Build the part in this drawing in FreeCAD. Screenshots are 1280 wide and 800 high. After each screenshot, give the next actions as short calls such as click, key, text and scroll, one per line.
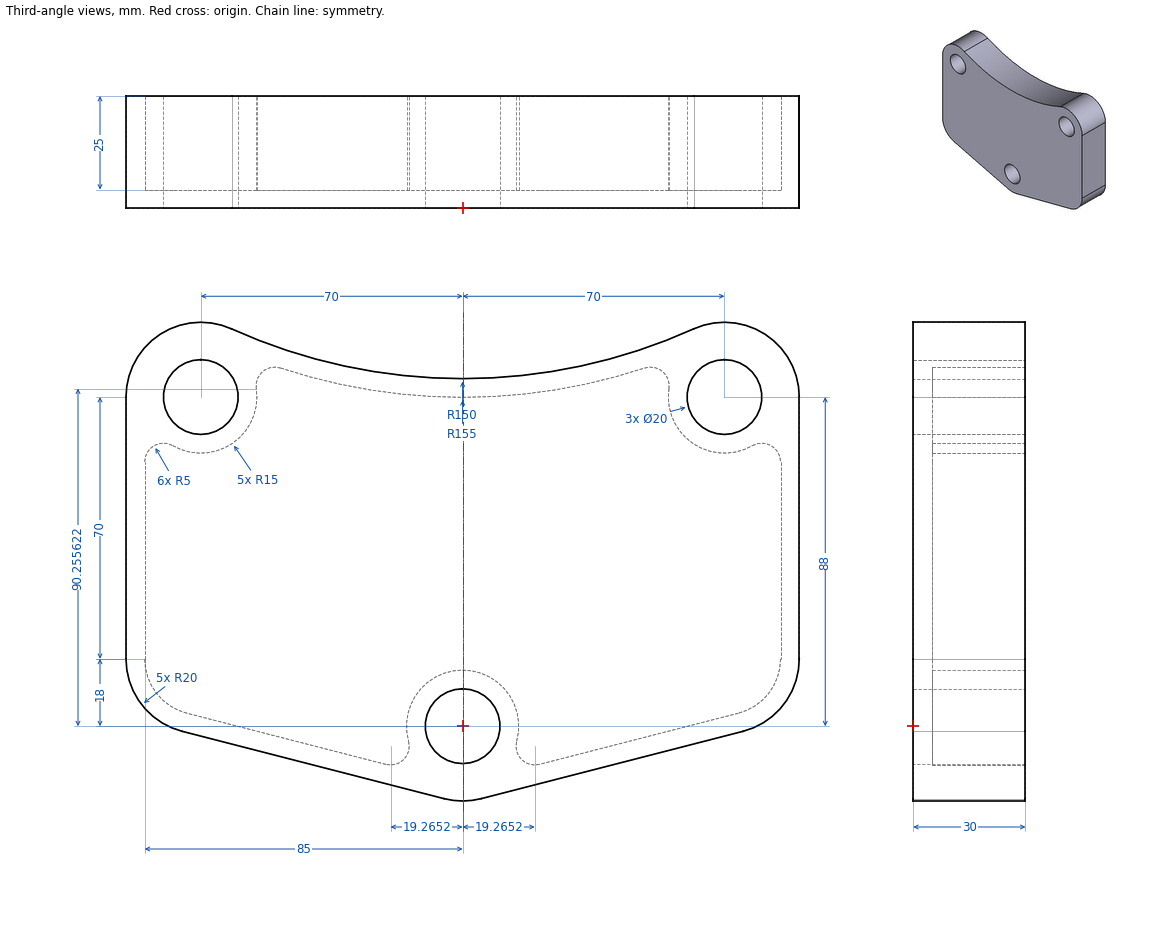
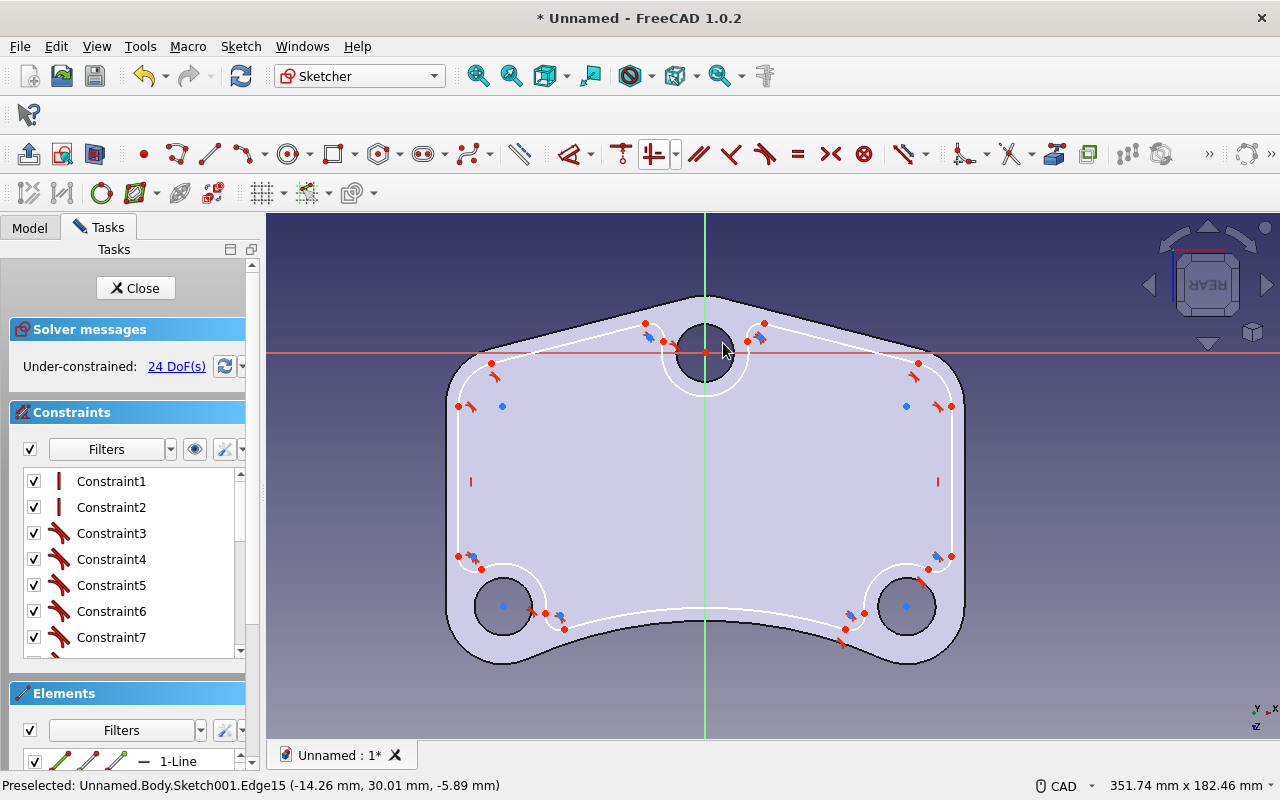
scroll(461, 565, up, 2)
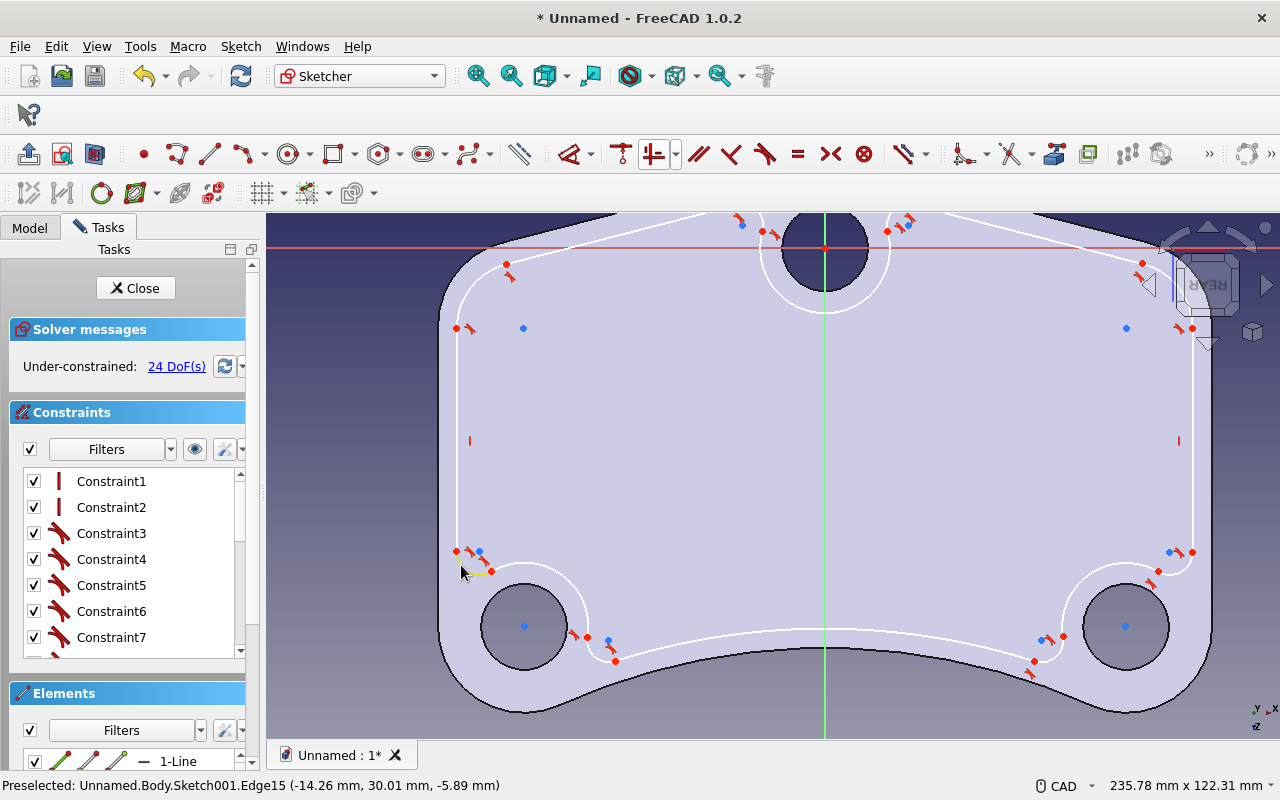
click(461, 565)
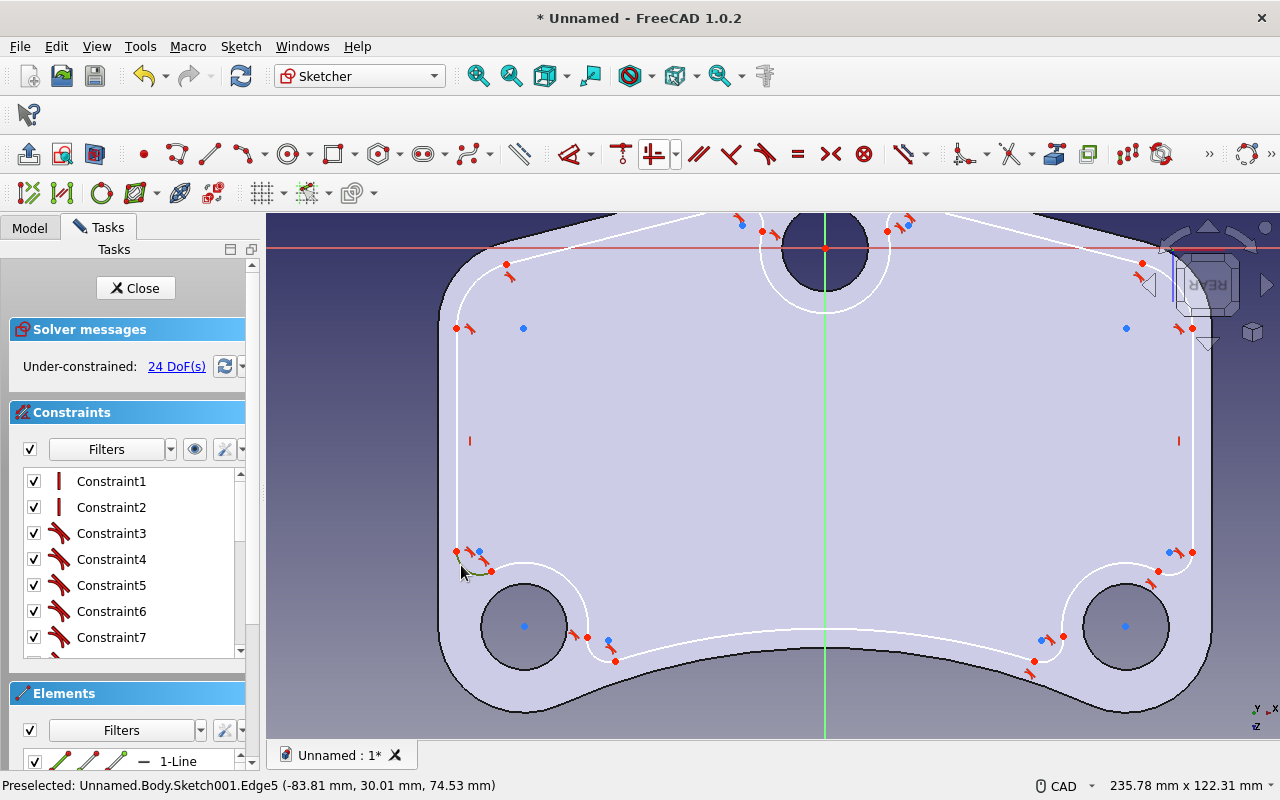
click(589, 650)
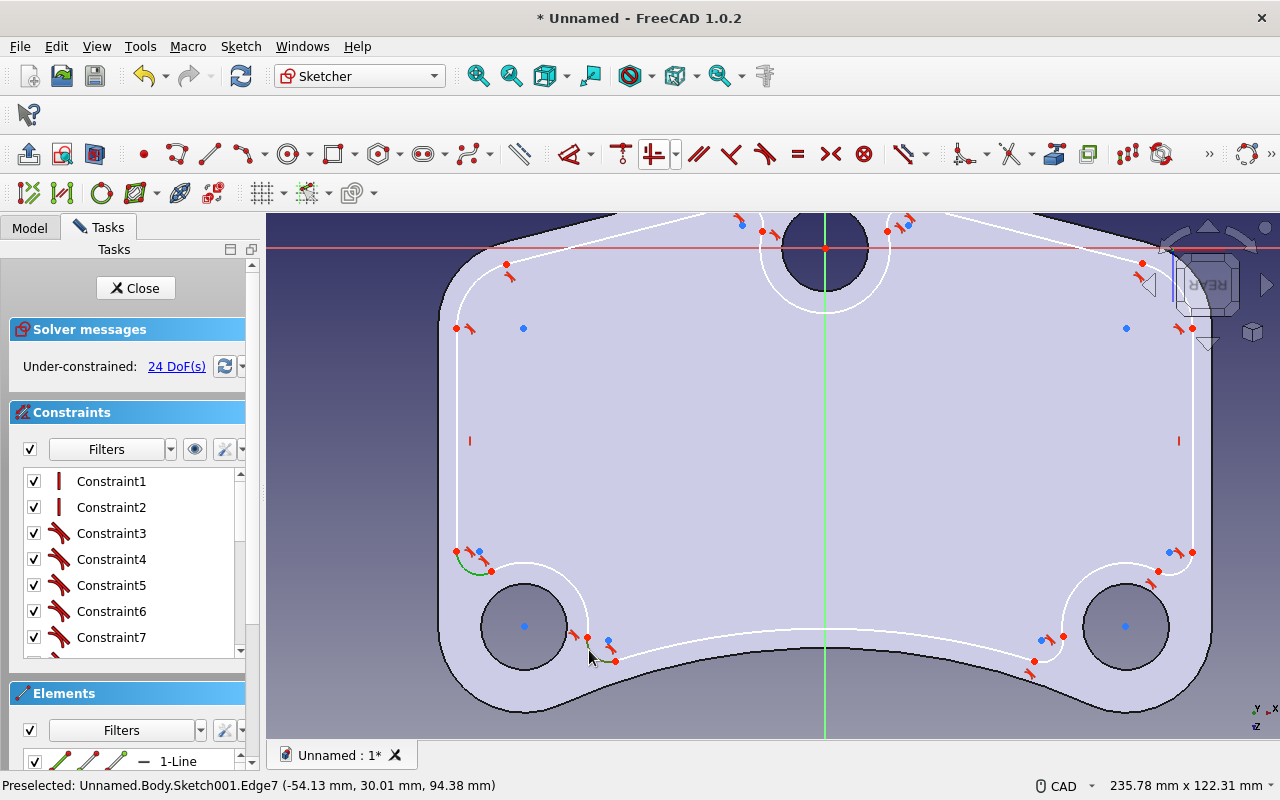
click(1048, 661)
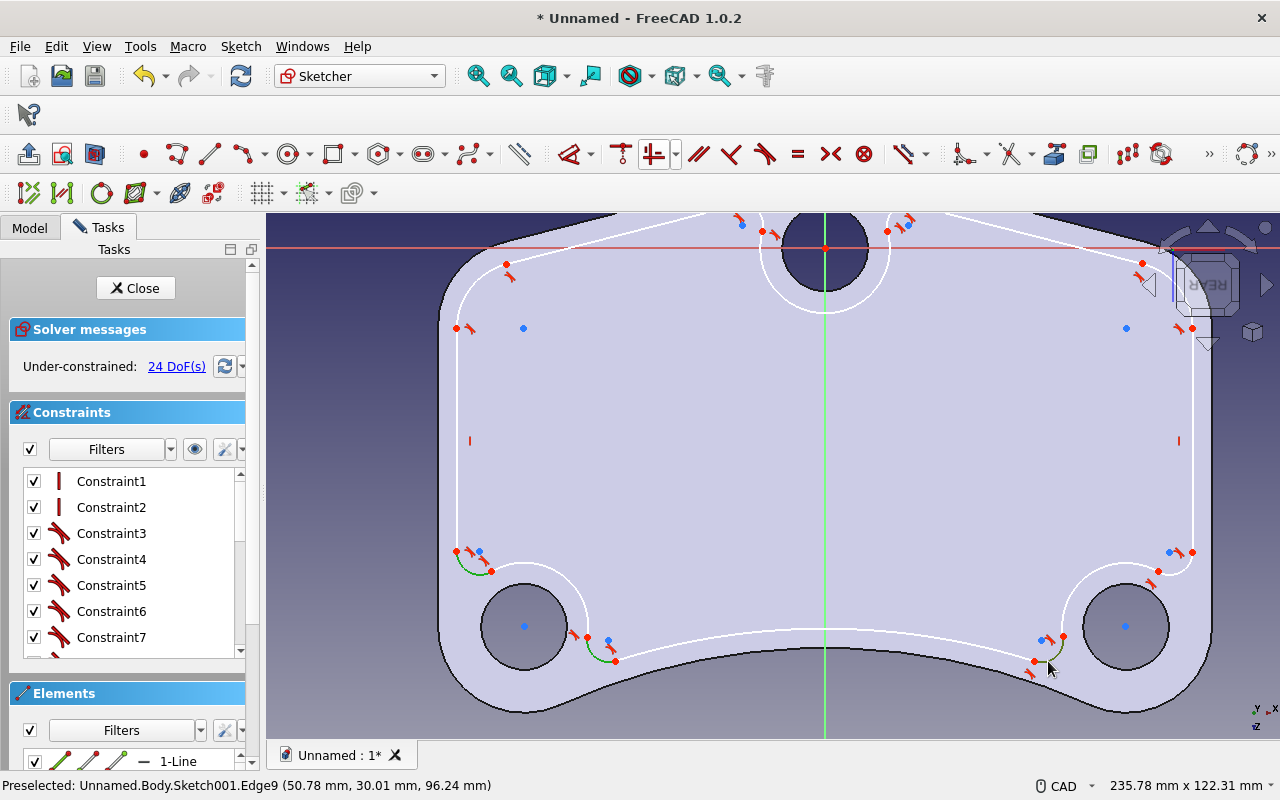
scroll(459, 565, down, 2)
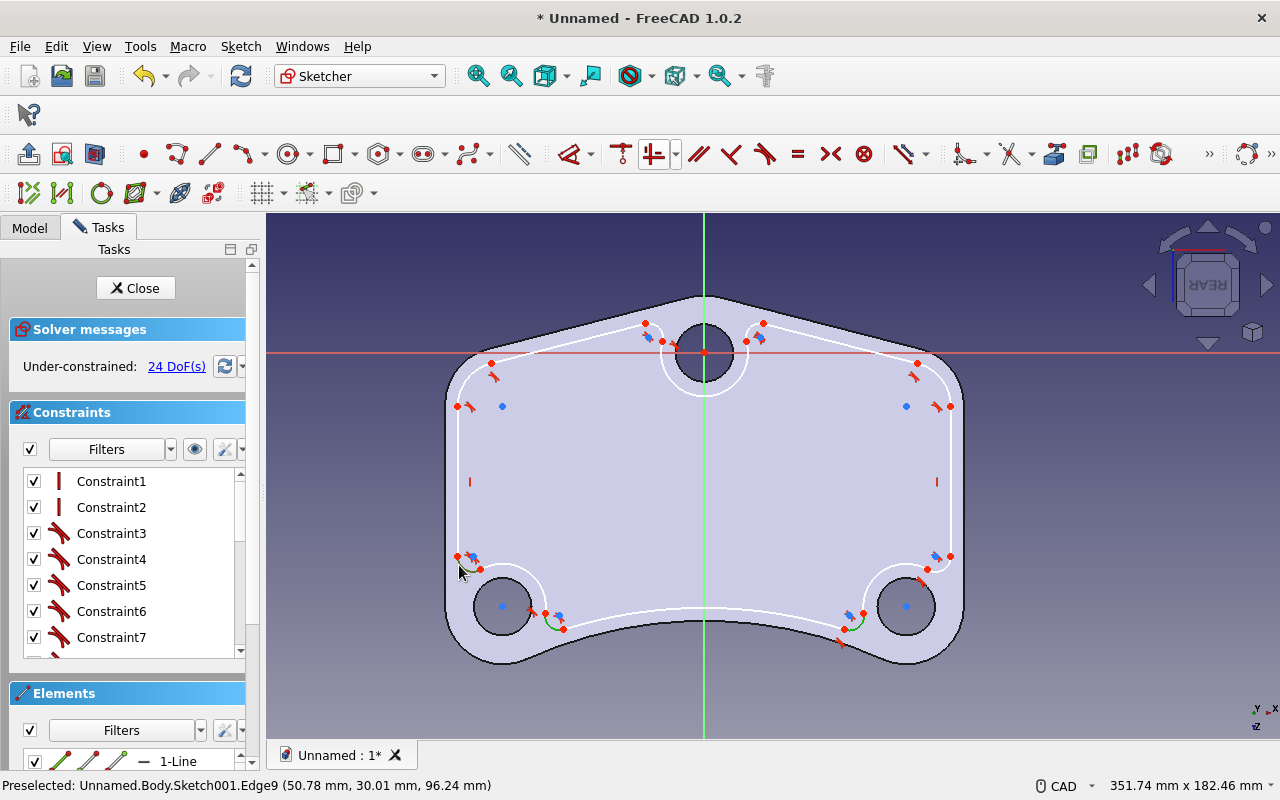
scroll(937, 572, up, 2)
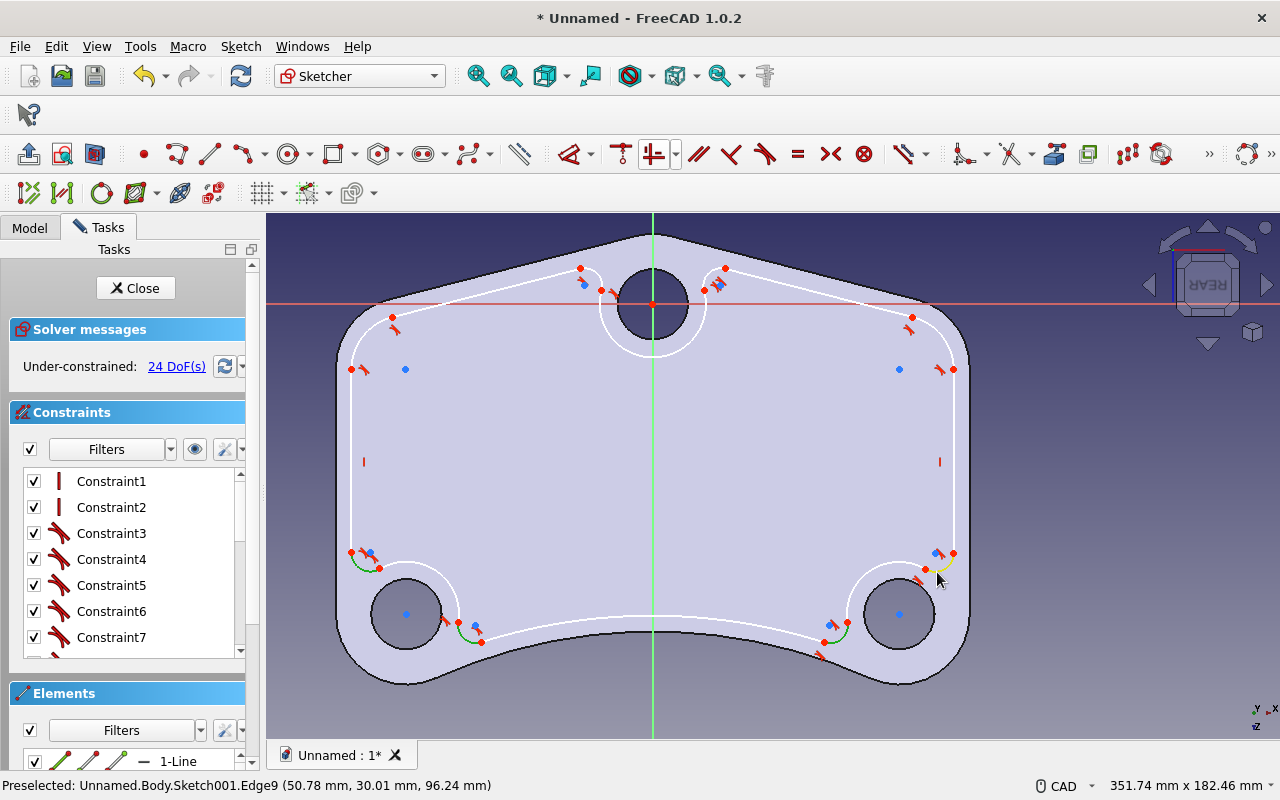
click(937, 571)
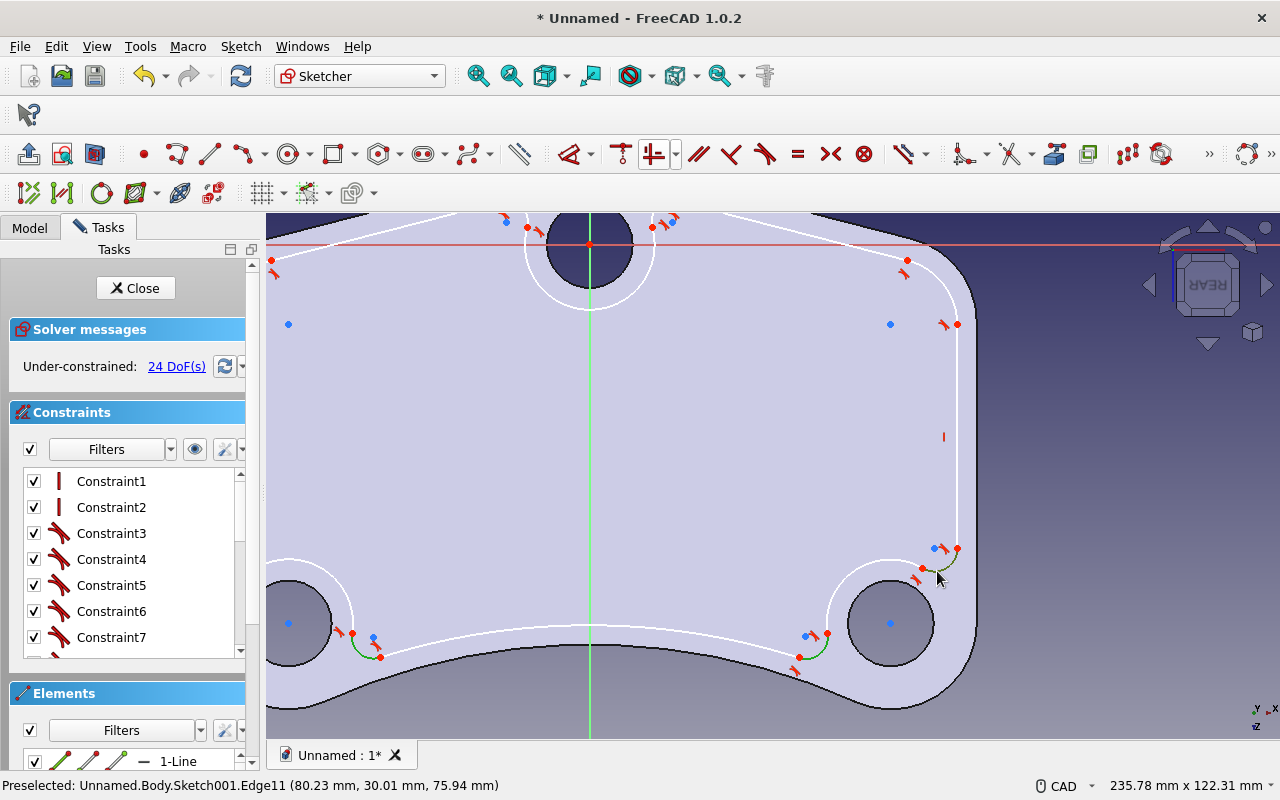
scroll(938, 572, down, 2)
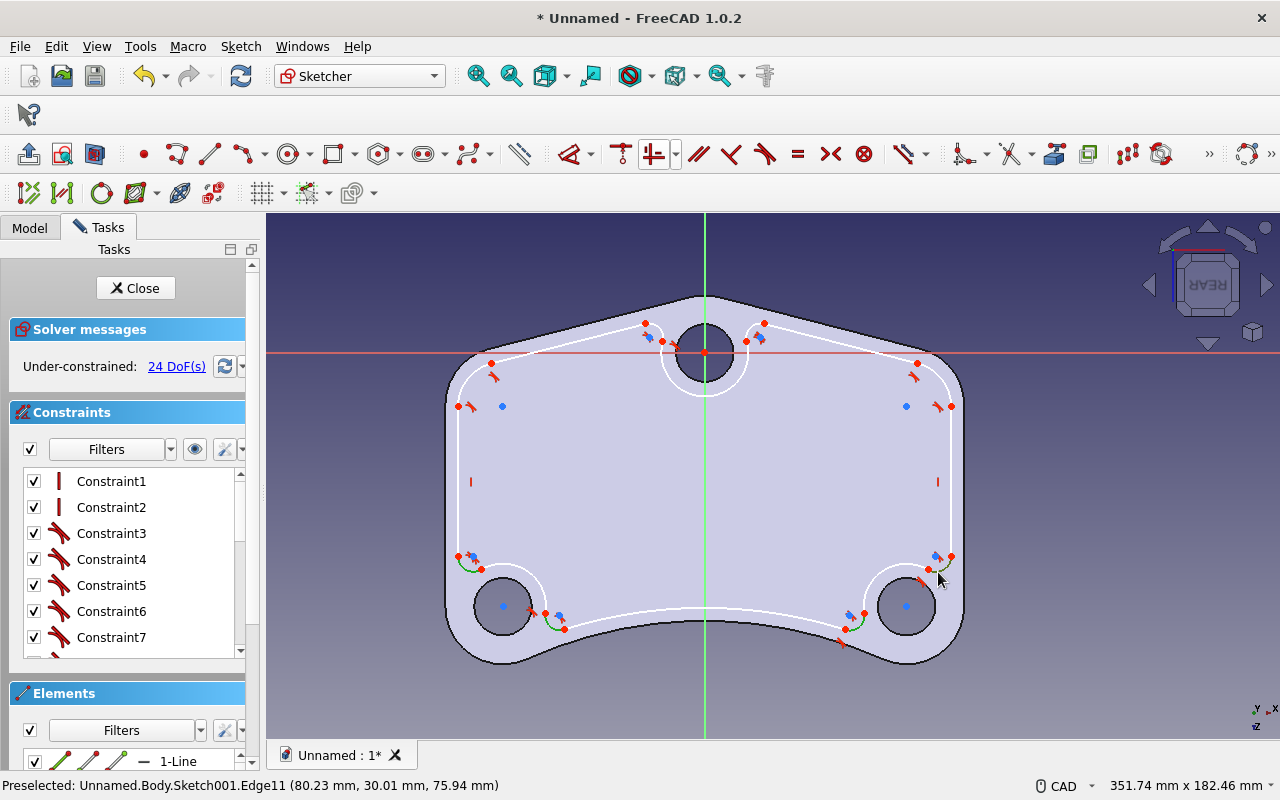
scroll(755, 324, up, 3)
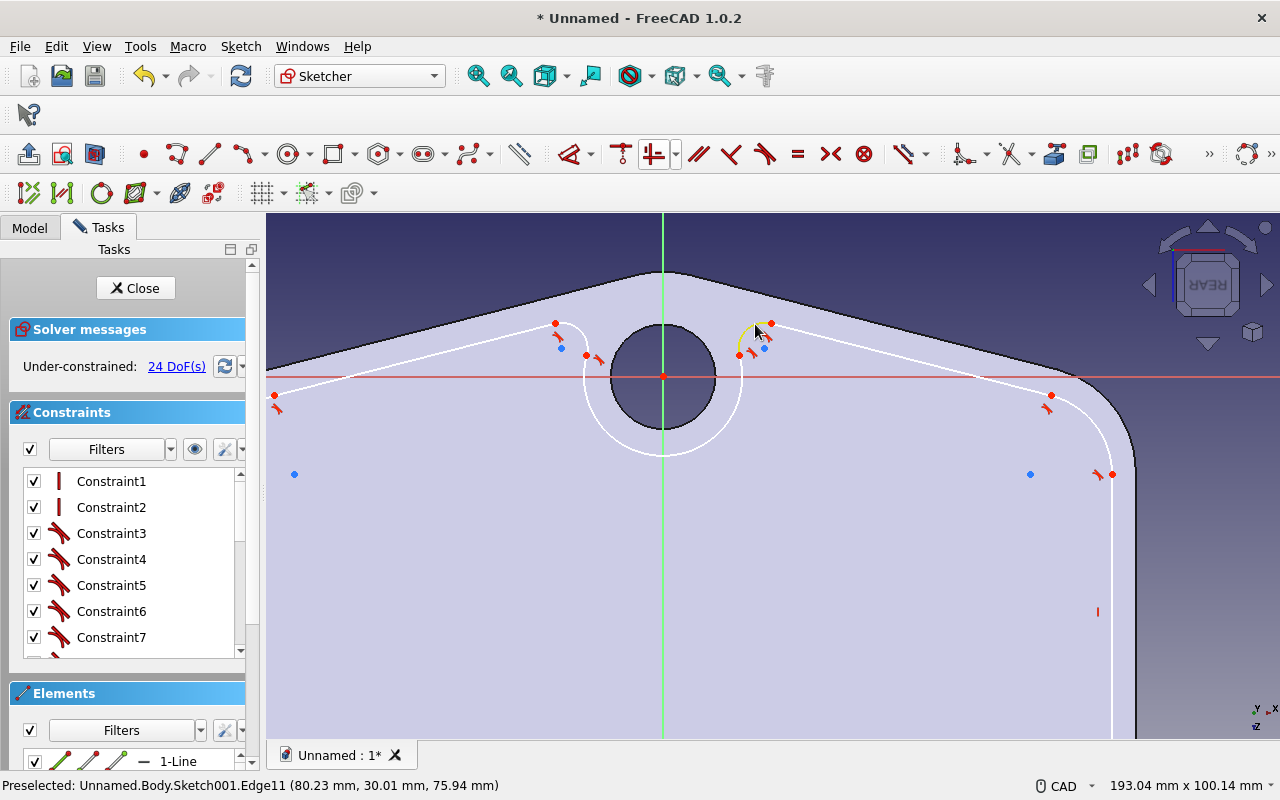
click(755, 325)